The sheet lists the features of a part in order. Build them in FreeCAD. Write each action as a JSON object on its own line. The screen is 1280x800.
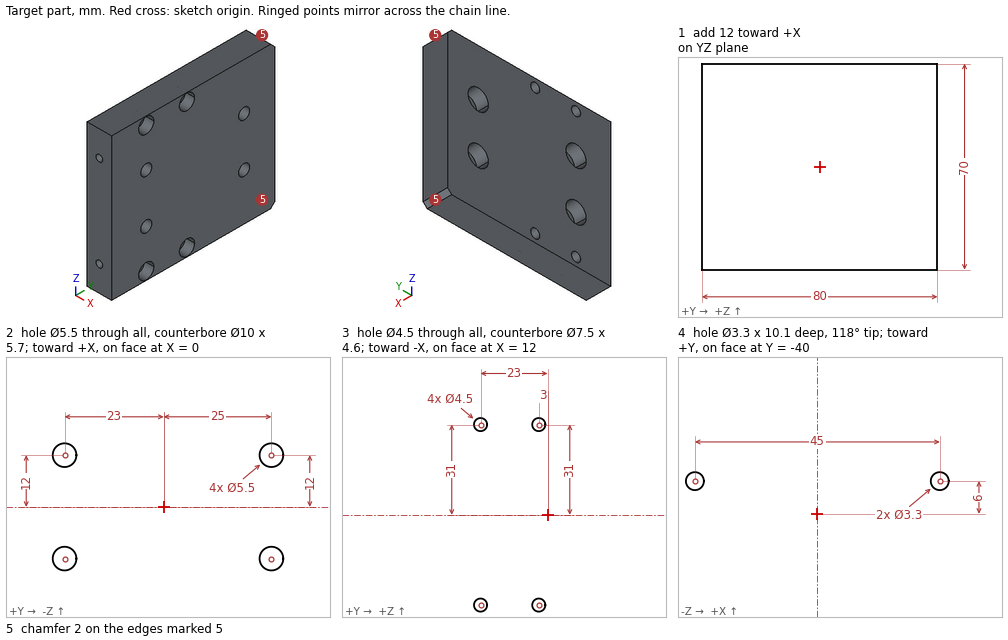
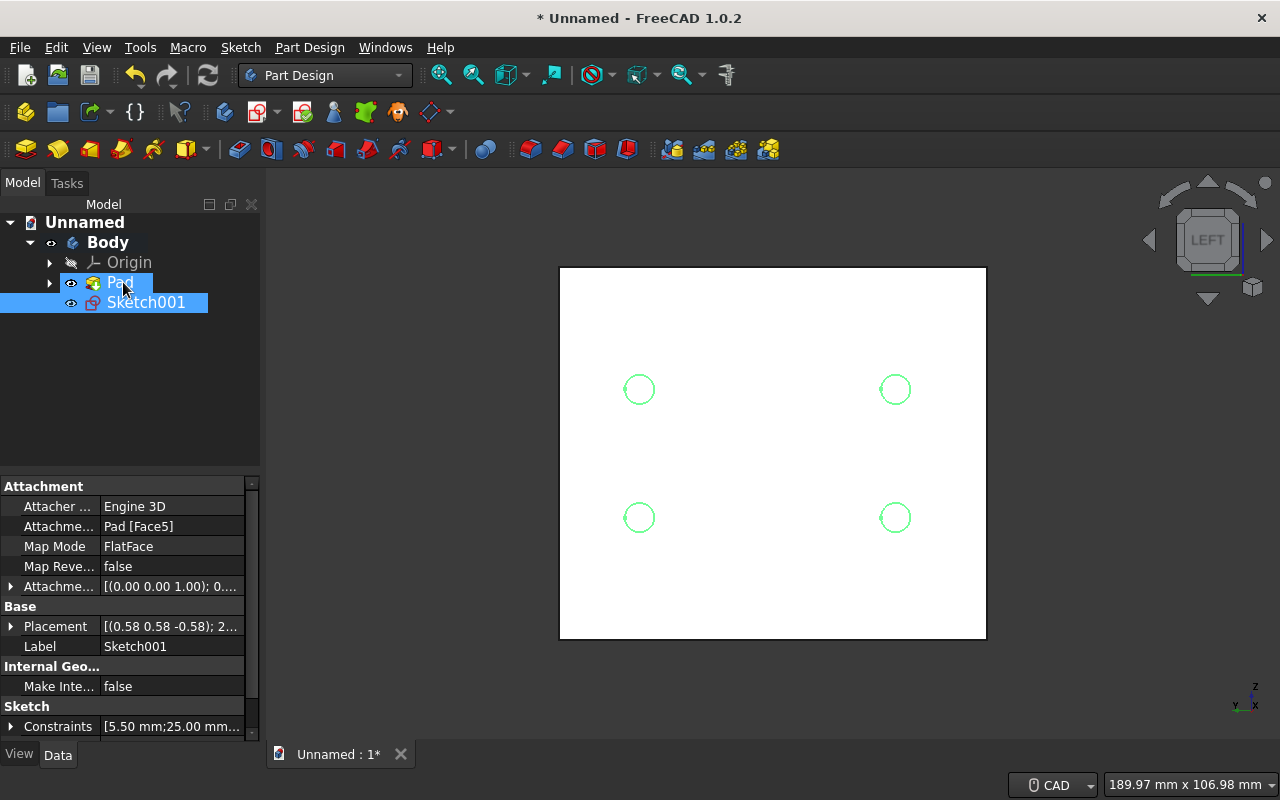
{"action": "left_click", "coordinate": [272, 150]}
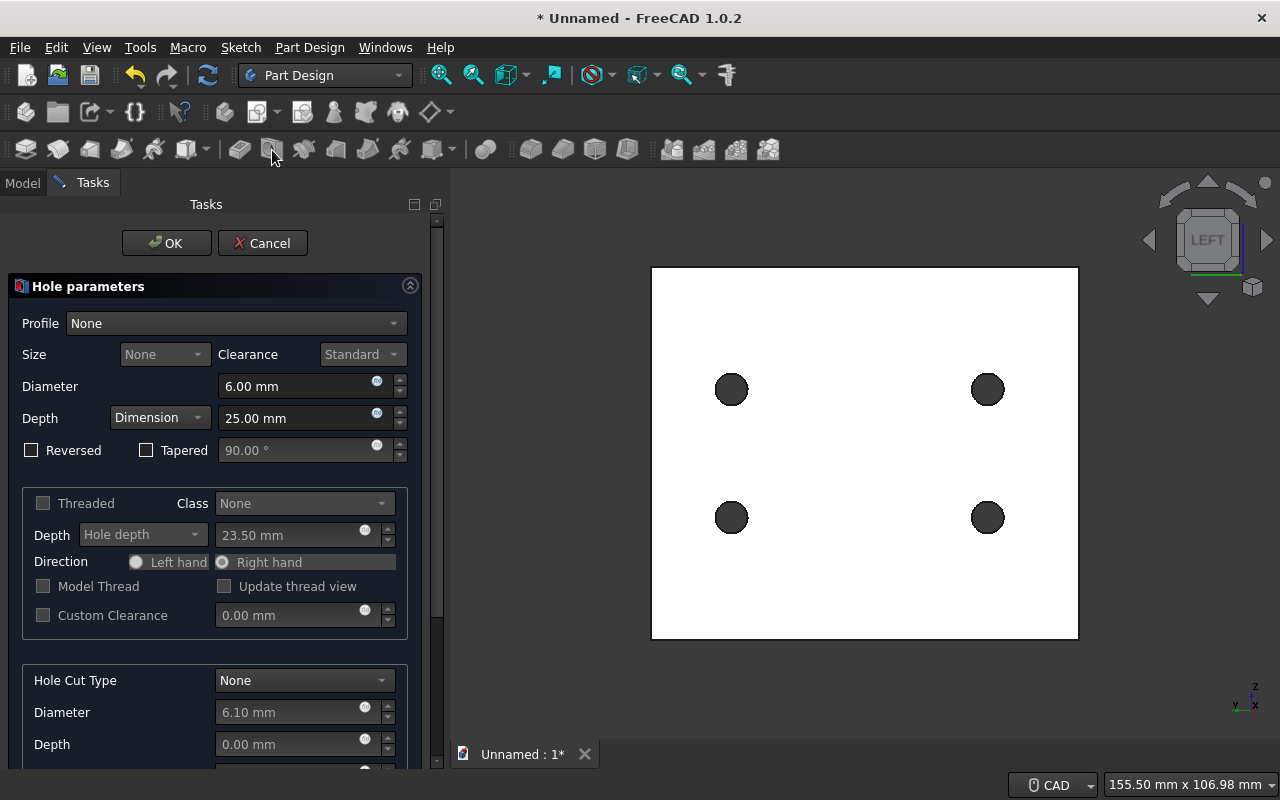
{"action": "triple_click", "coordinate": [305, 386]}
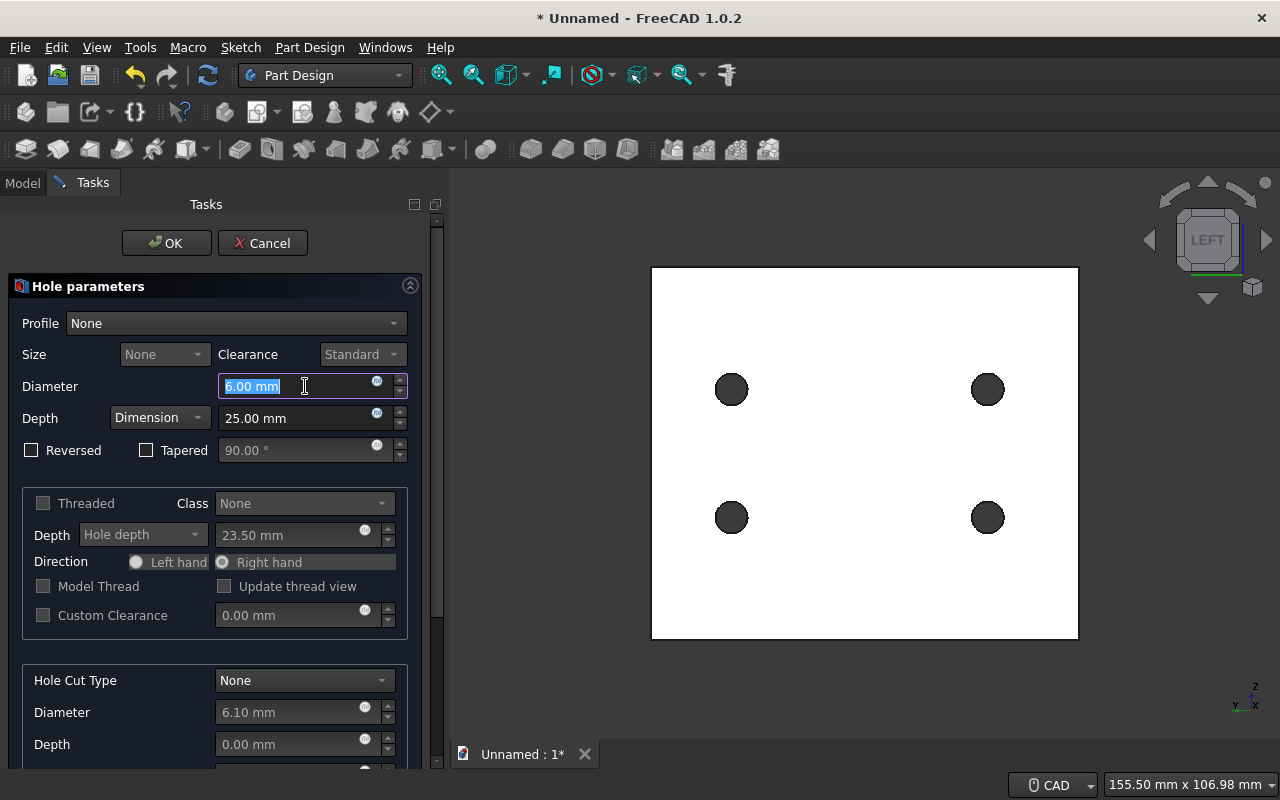
{"action": "type", "text": "5.5"}
{"action": "key", "text": "Tab"}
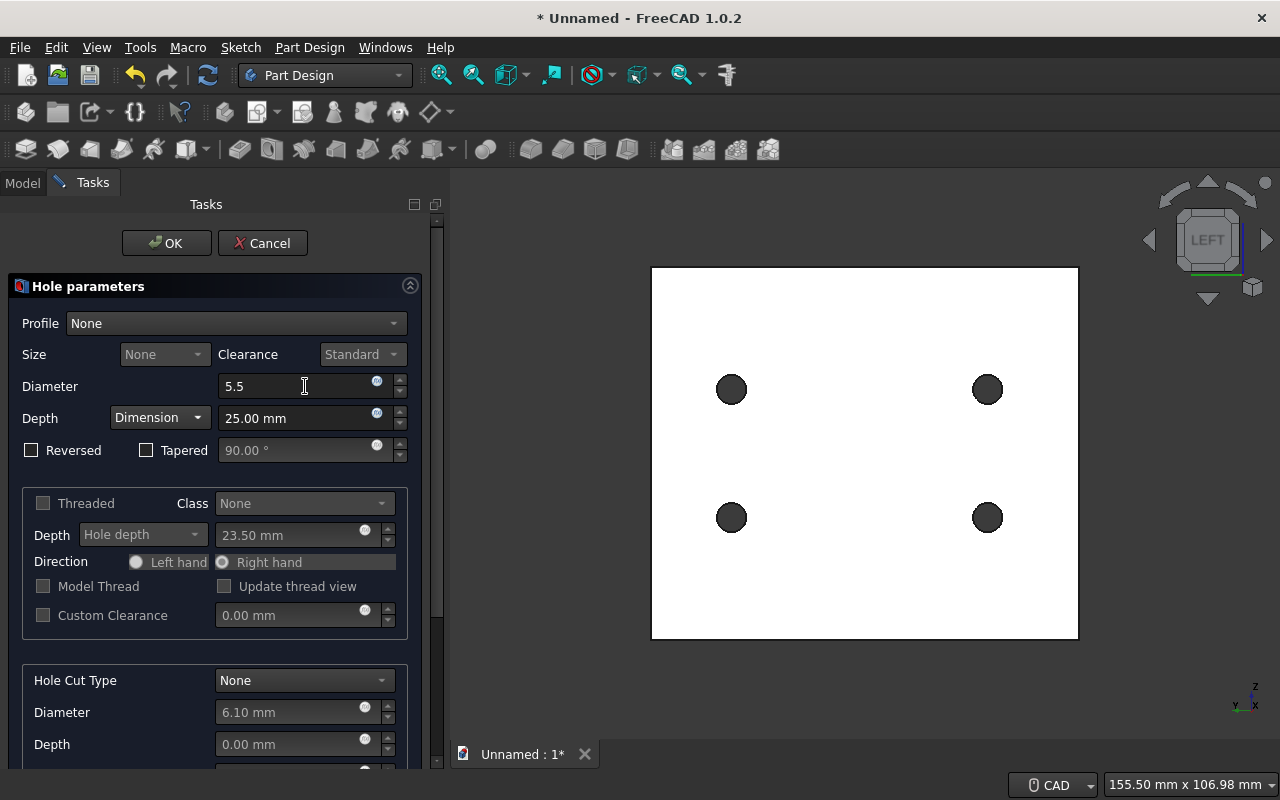
{"action": "left_click", "coordinate": [161, 418]}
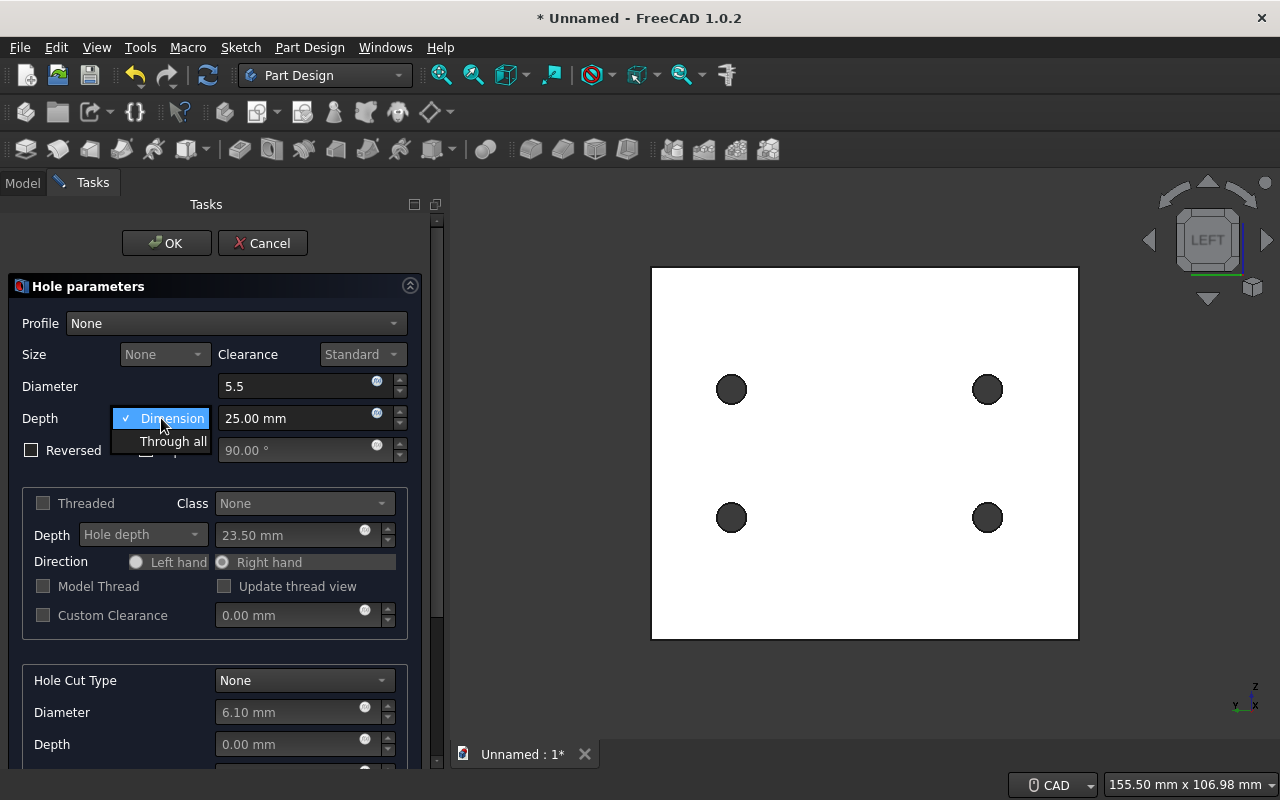
{"action": "left_click", "coordinate": [160, 442]}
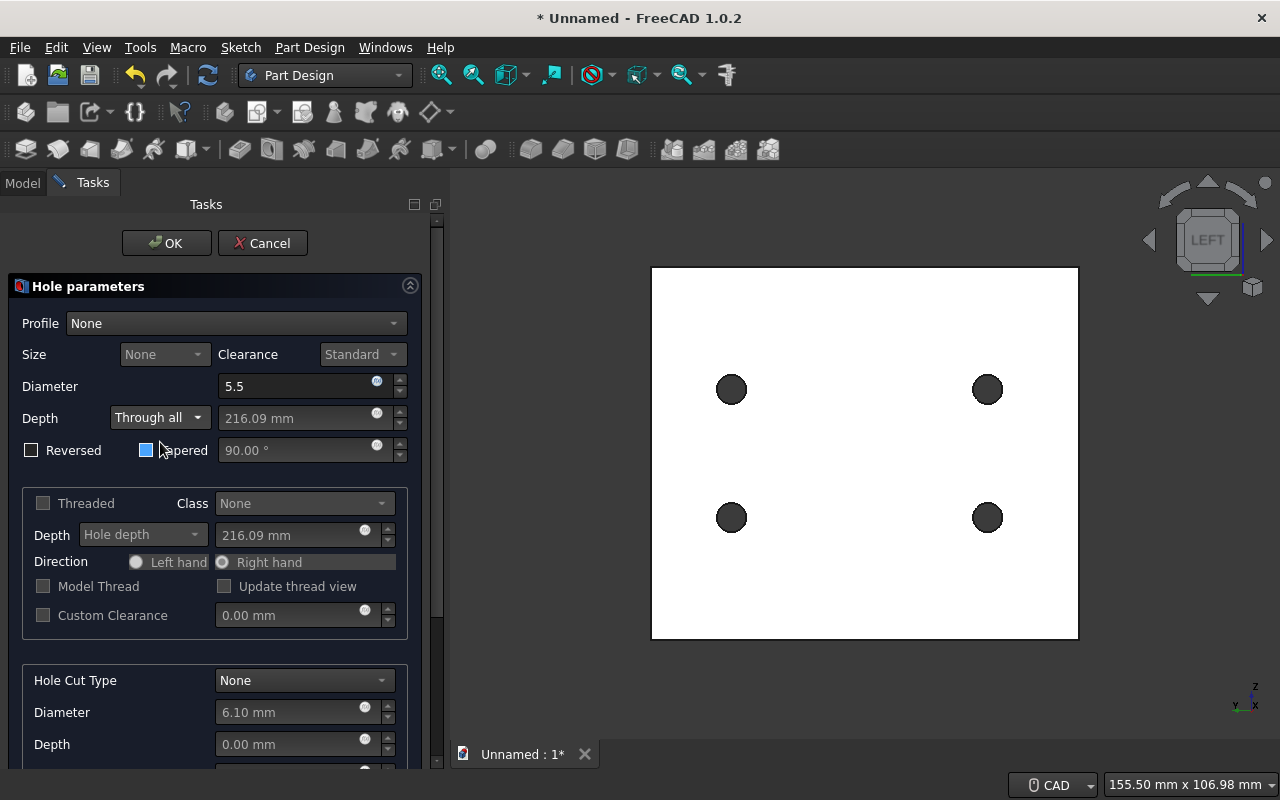
{"action": "left_click", "coordinate": [306, 680]}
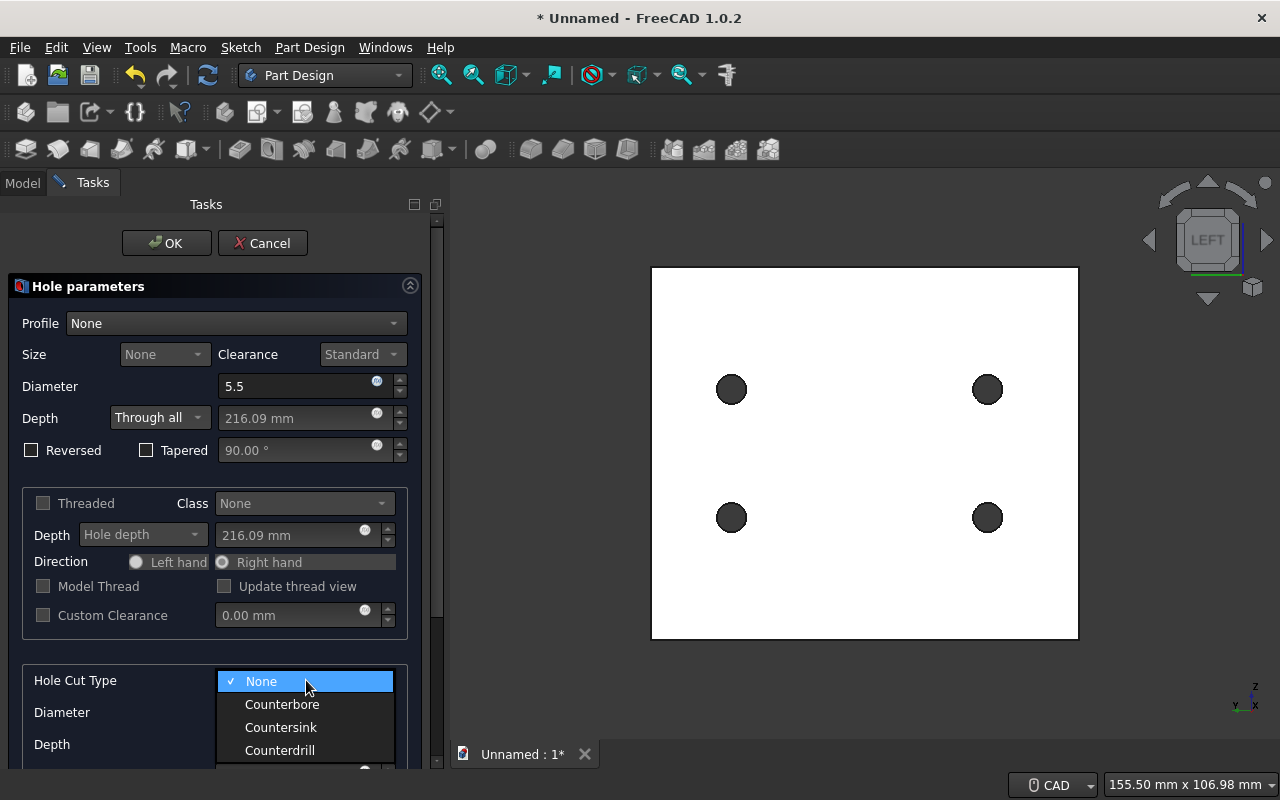
{"action": "left_click", "coordinate": [304, 704]}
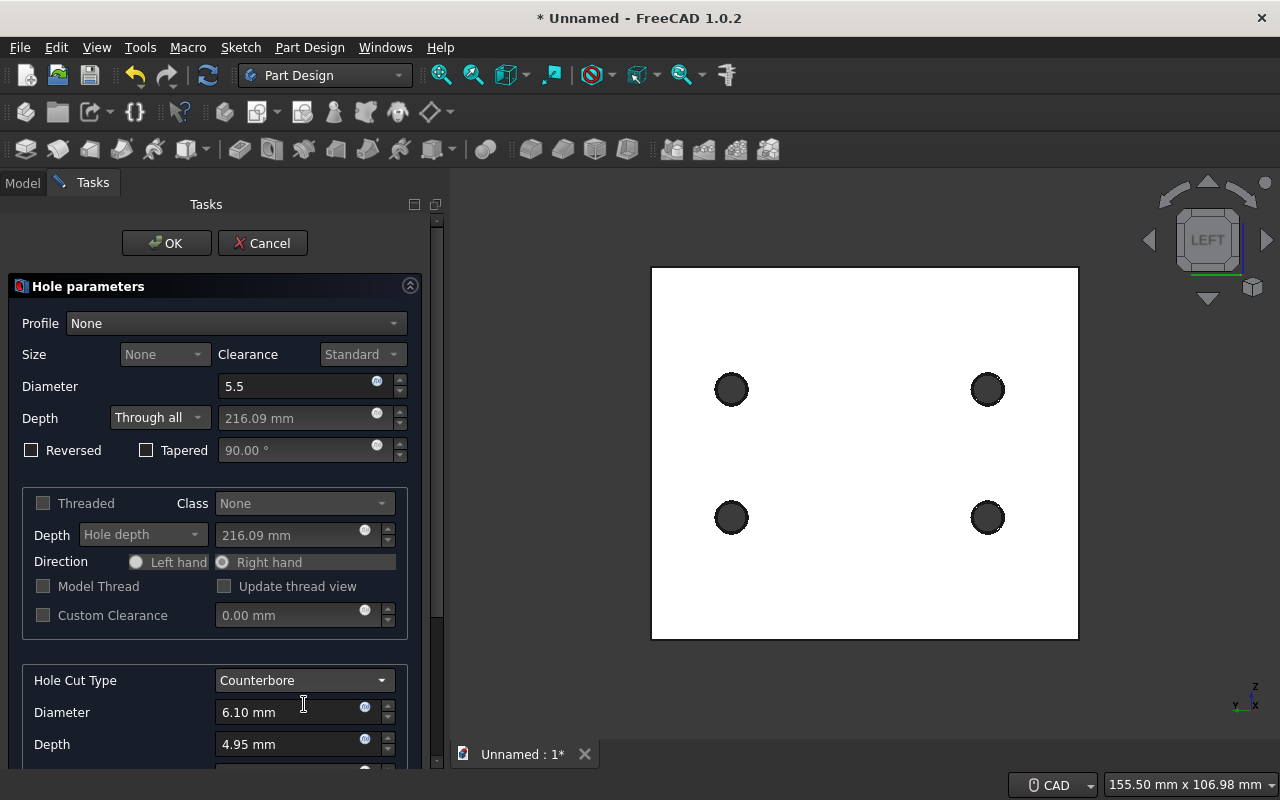
{"action": "triple_click", "coordinate": [298, 712]}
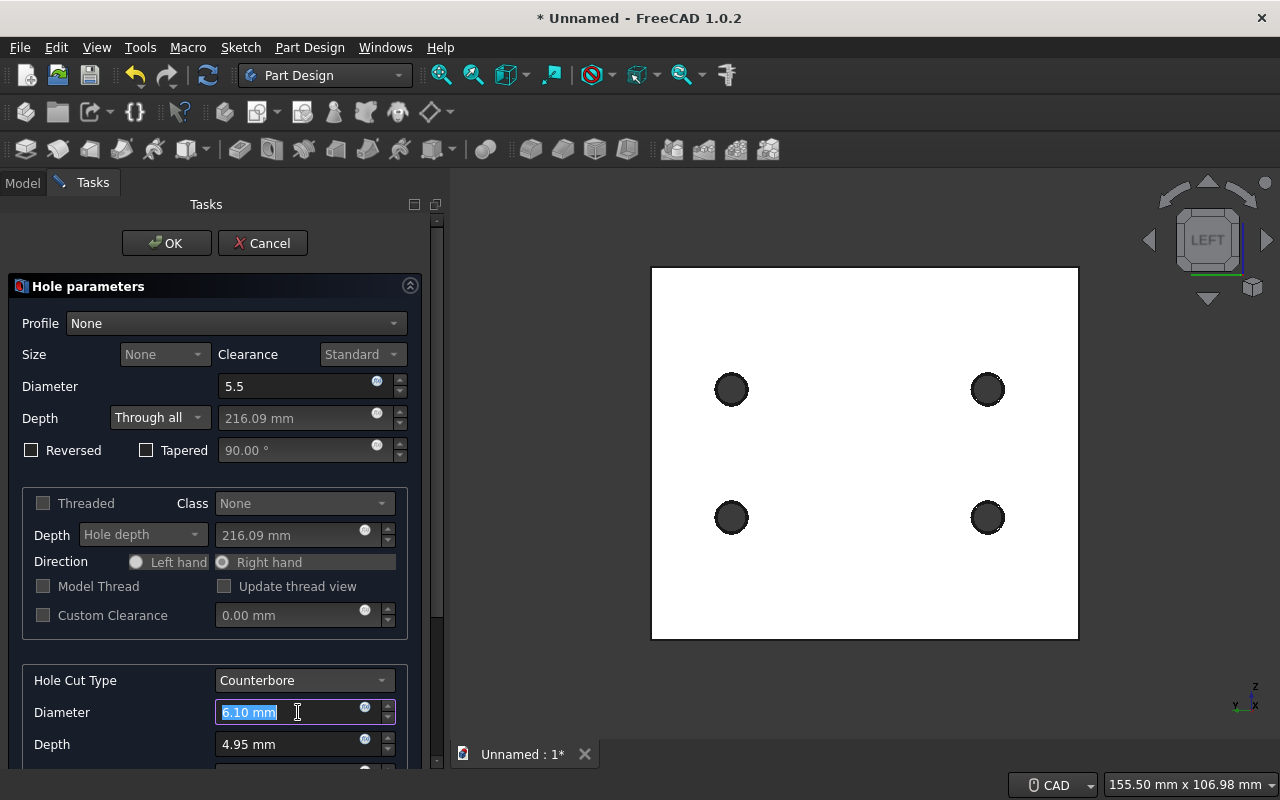
{"action": "type", "text": "10"}
{"action": "key", "text": "Tab"}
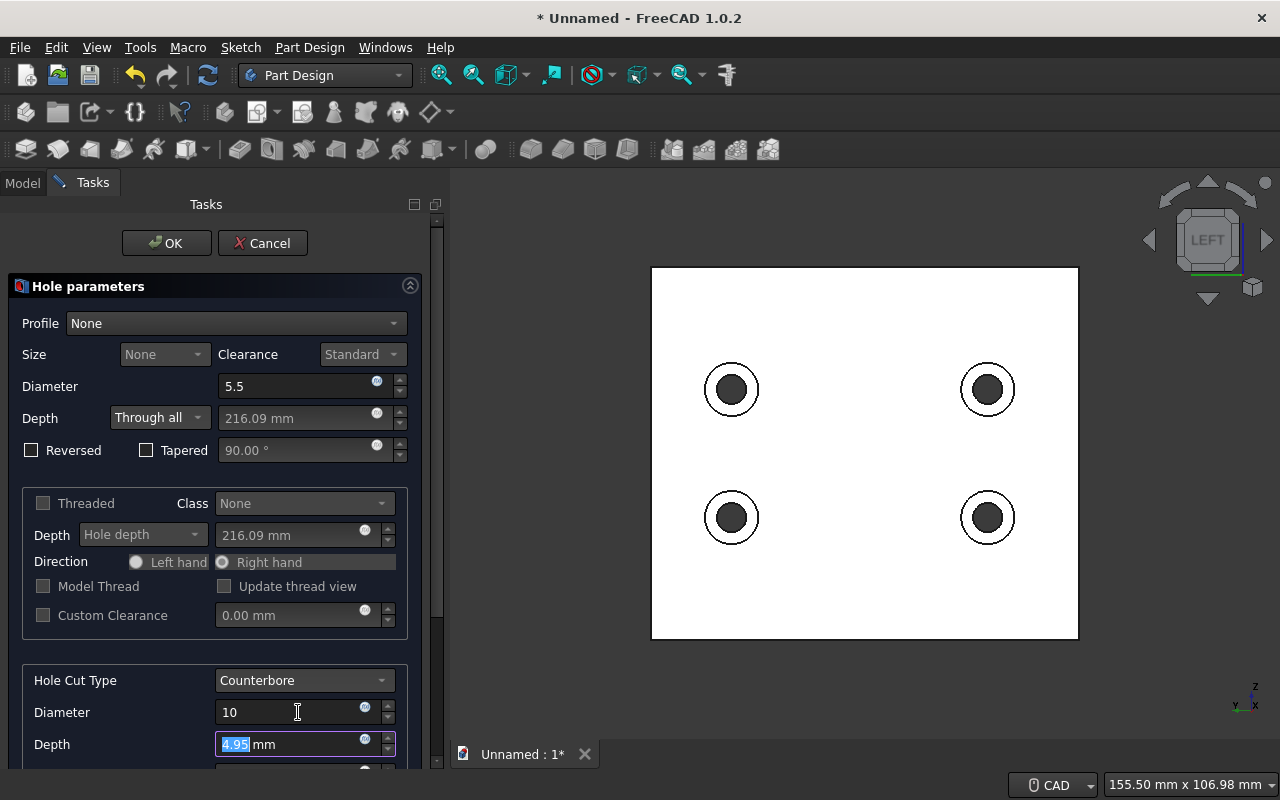
{"action": "type", "text": "5.7"}
{"action": "key", "text": "Tab"}